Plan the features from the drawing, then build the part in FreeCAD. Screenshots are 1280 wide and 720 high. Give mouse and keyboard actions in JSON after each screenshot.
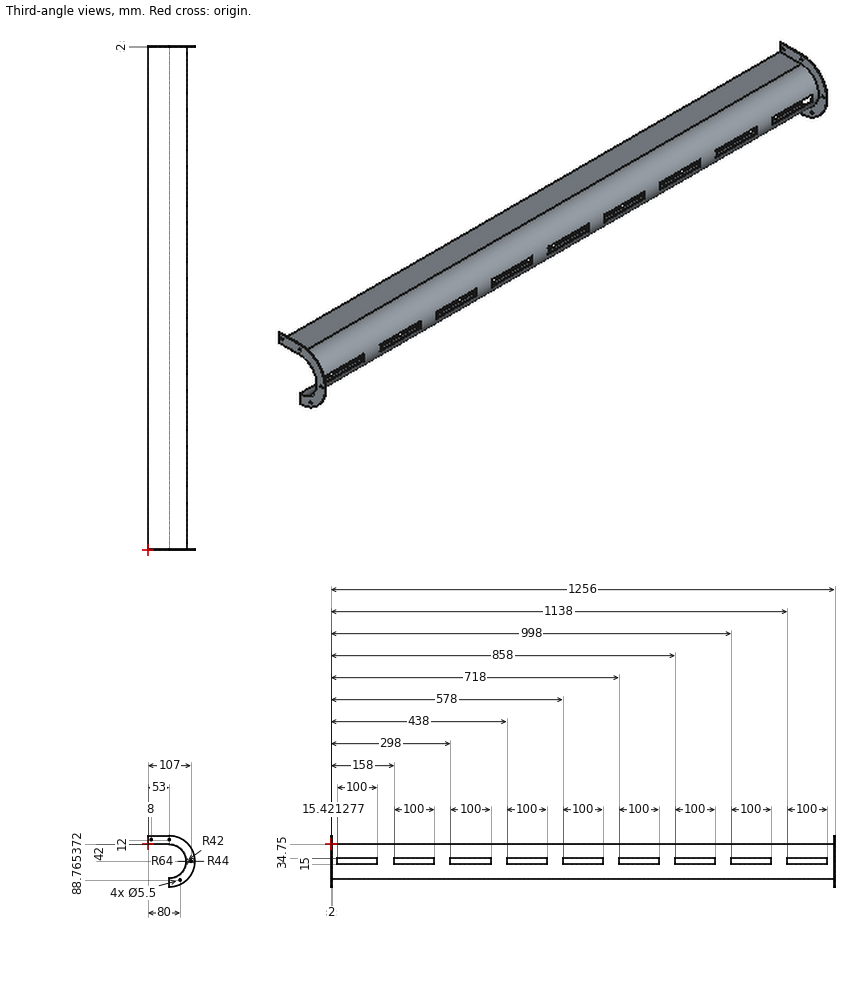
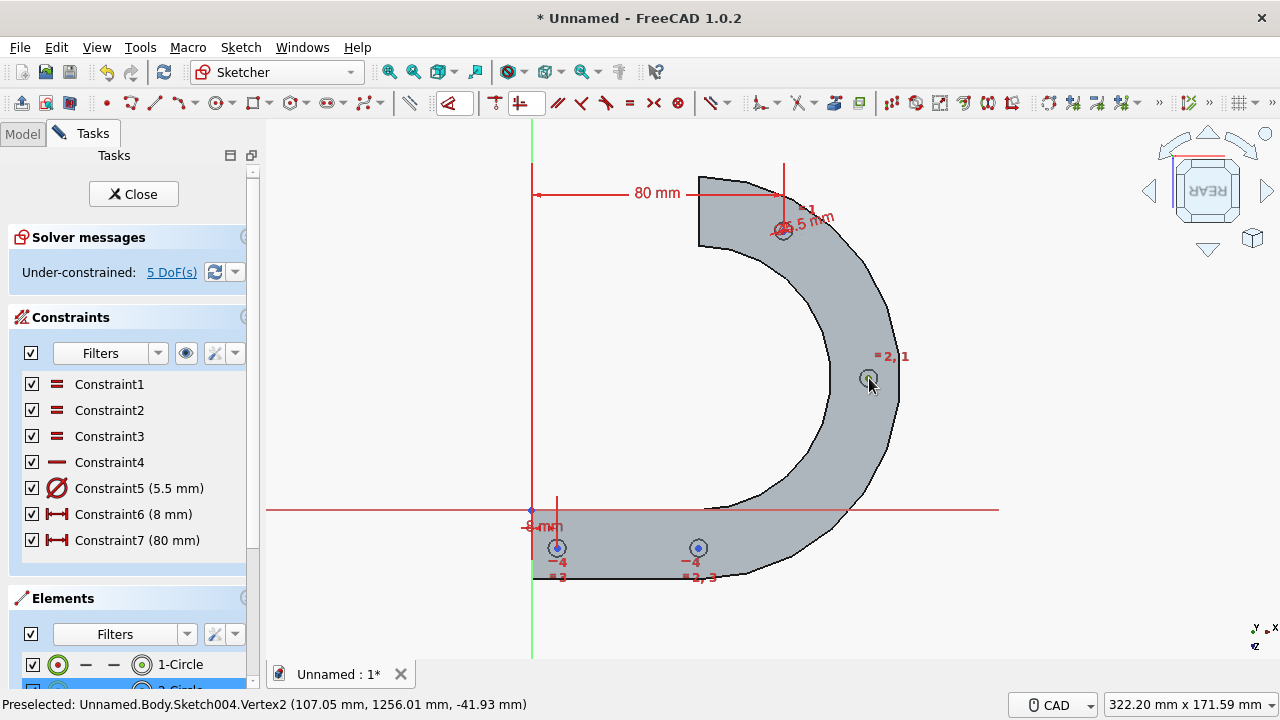
{"action": "key", "text": "i"}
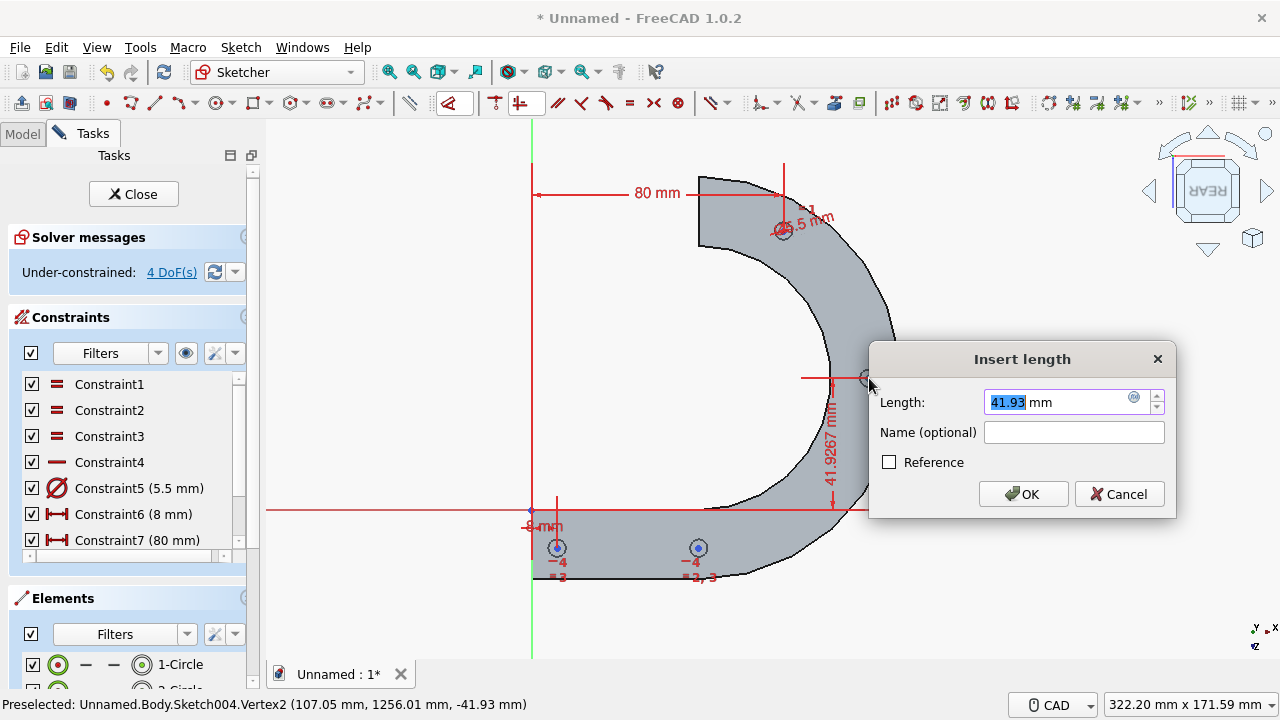
{"action": "type", "text": "42"}
{"action": "key", "text": "Return"}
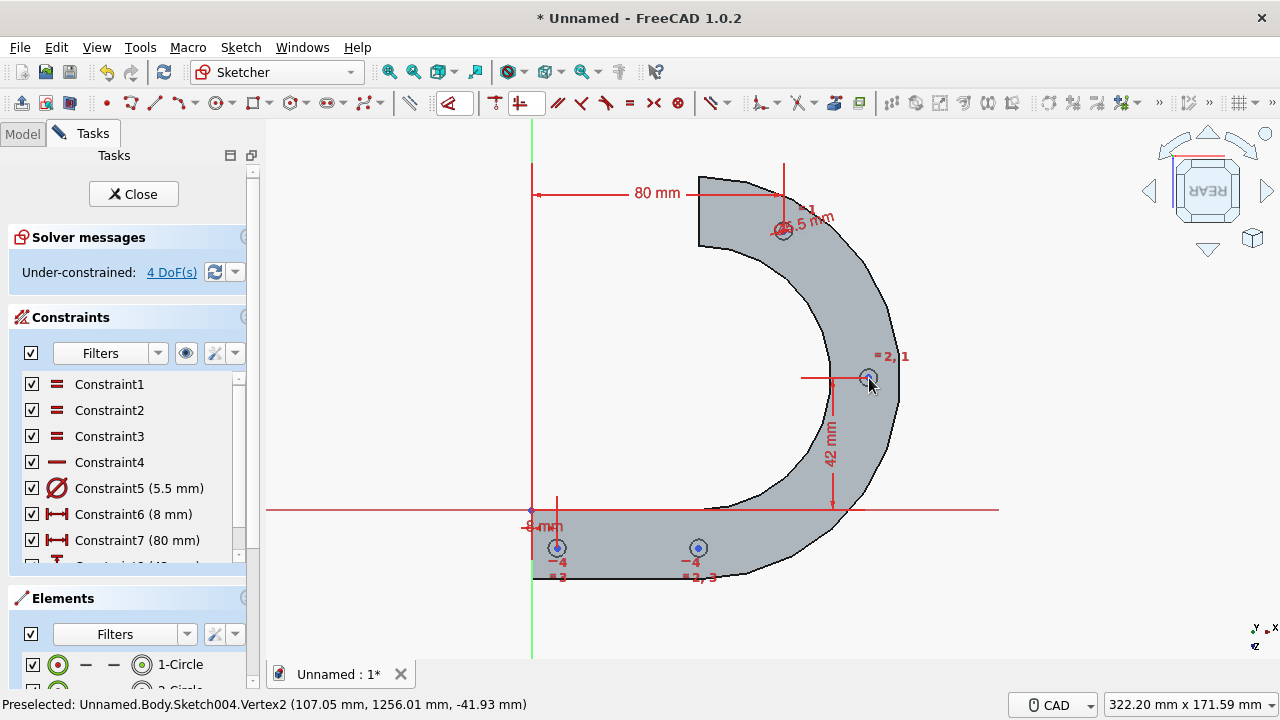
{"action": "left_click", "coordinate": [699, 548]}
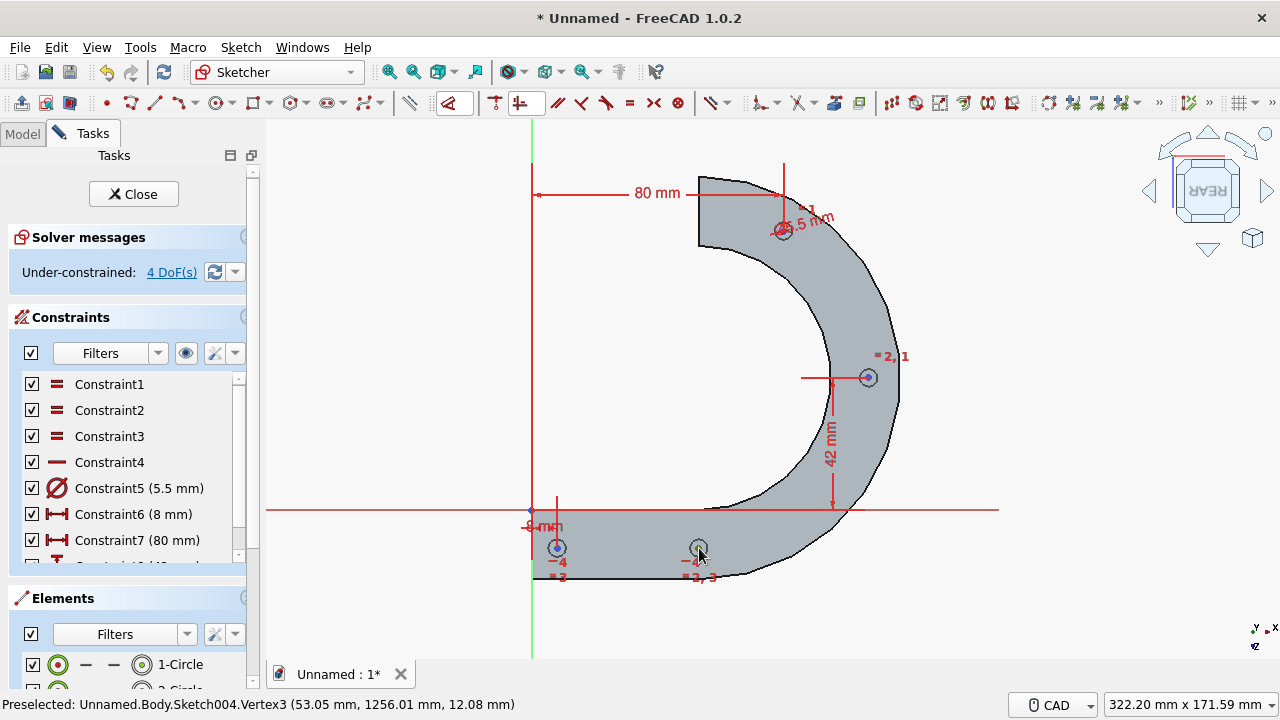
{"action": "left_click", "coordinate": [468, 104]}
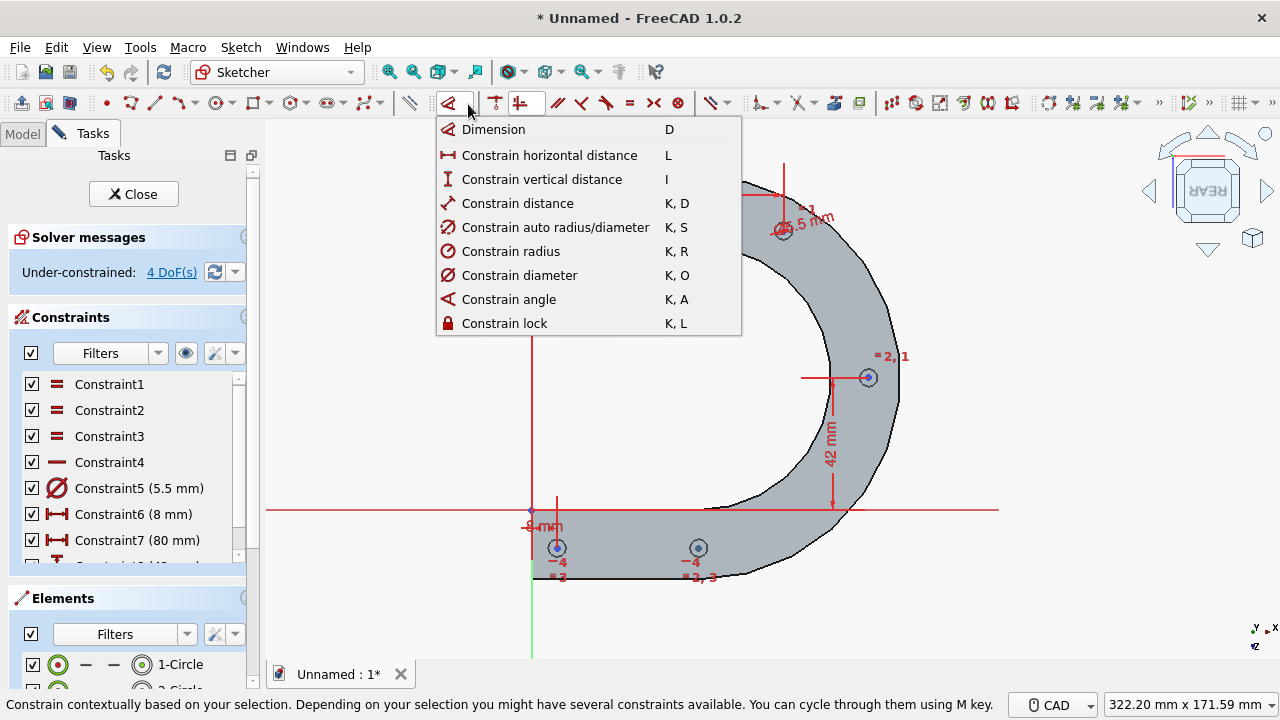
{"action": "left_click", "coordinate": [589, 155]}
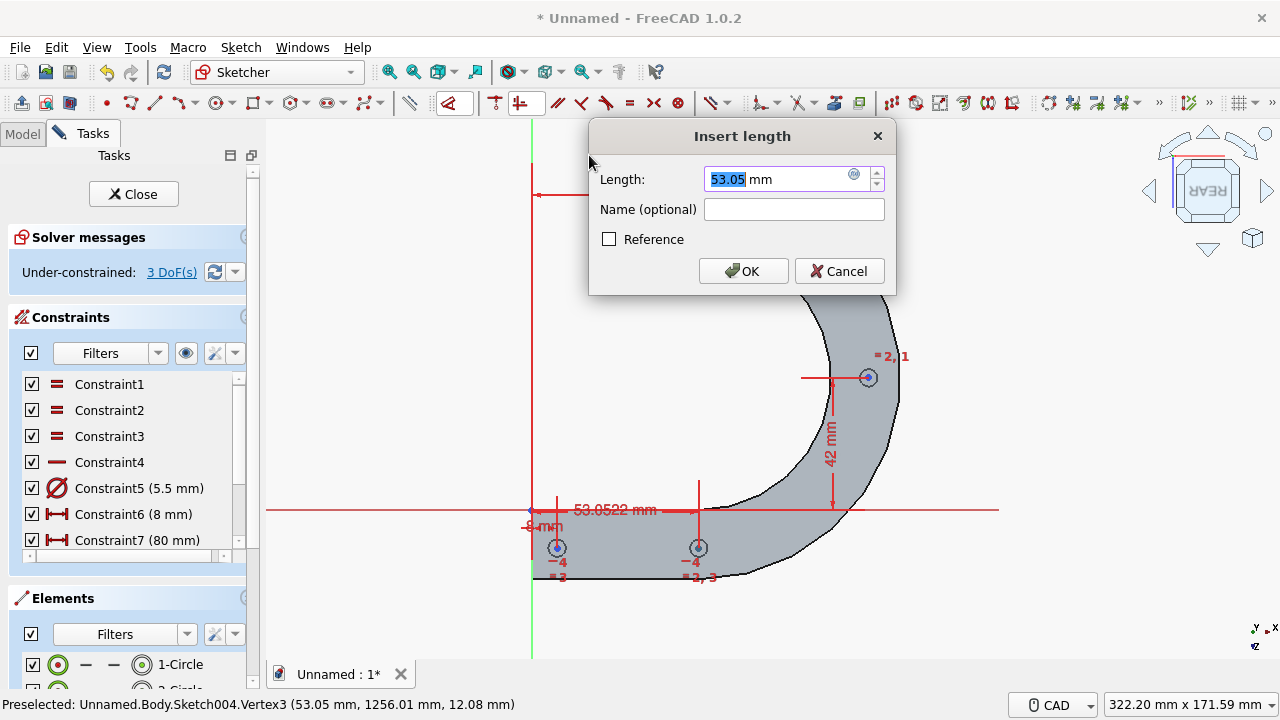
{"action": "type", "text": "53"}
{"action": "key", "text": "Return"}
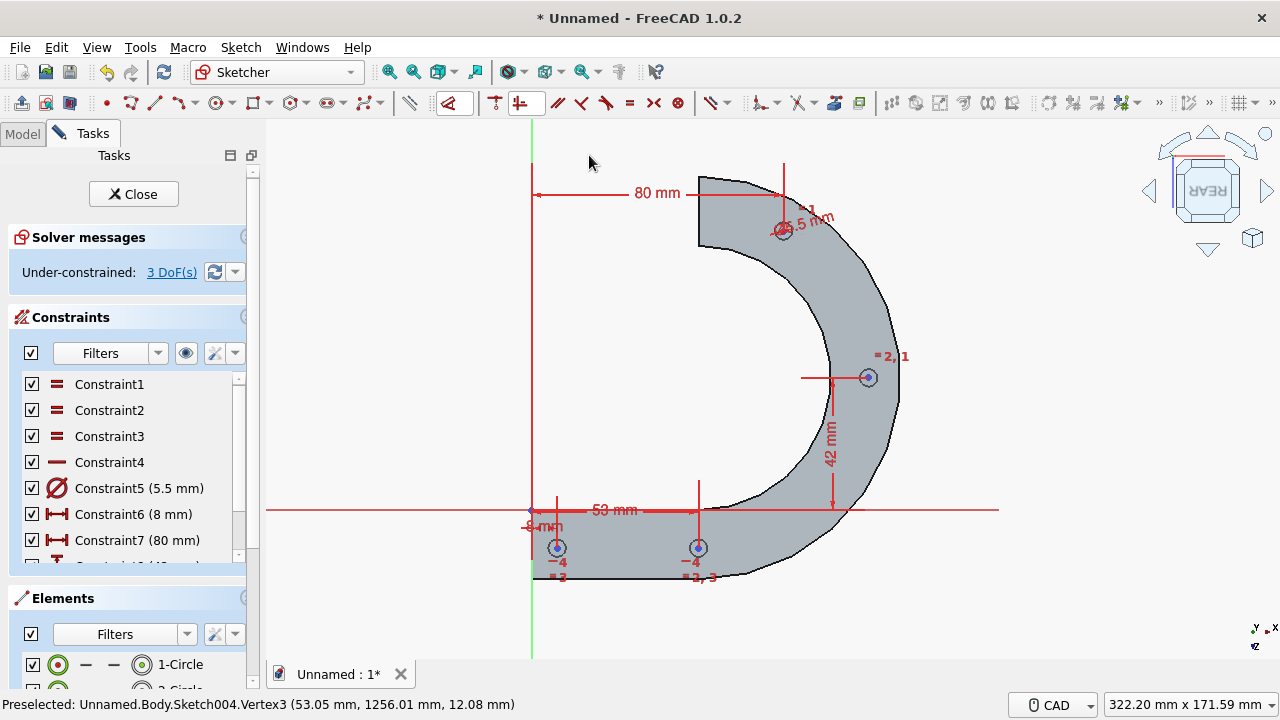
{"action": "left_click", "coordinate": [699, 548]}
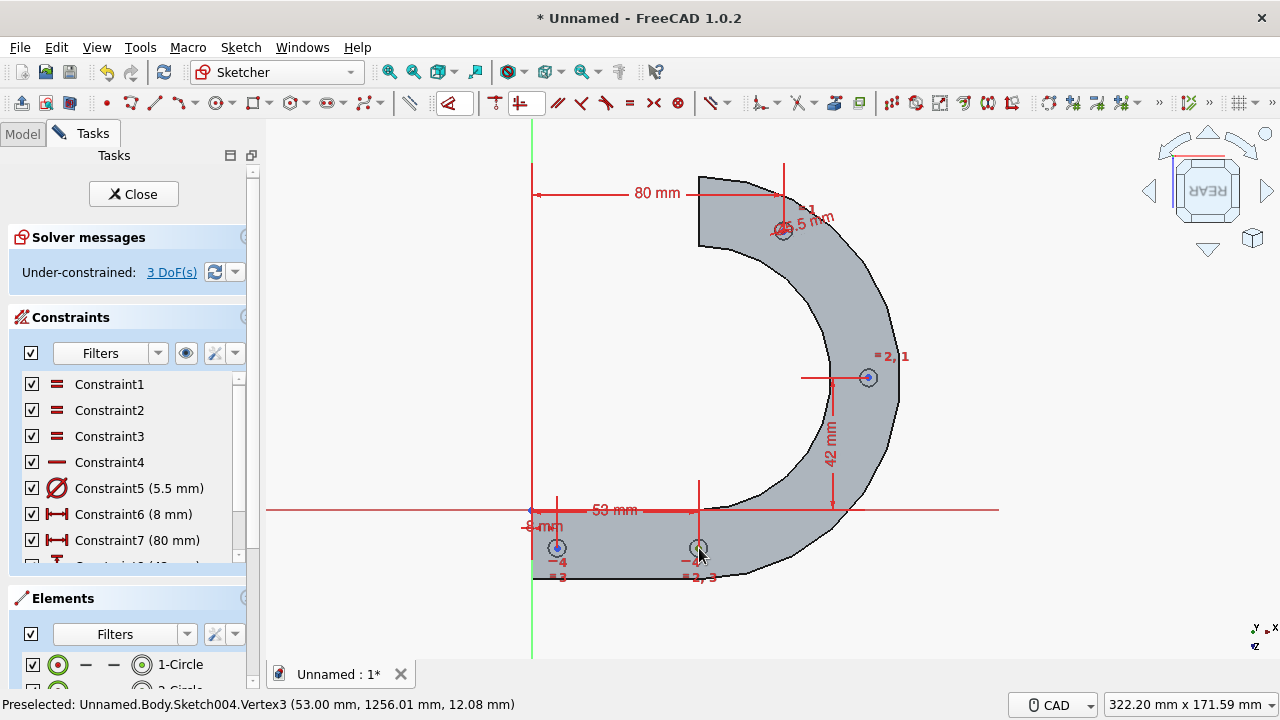
{"action": "key", "text": "i"}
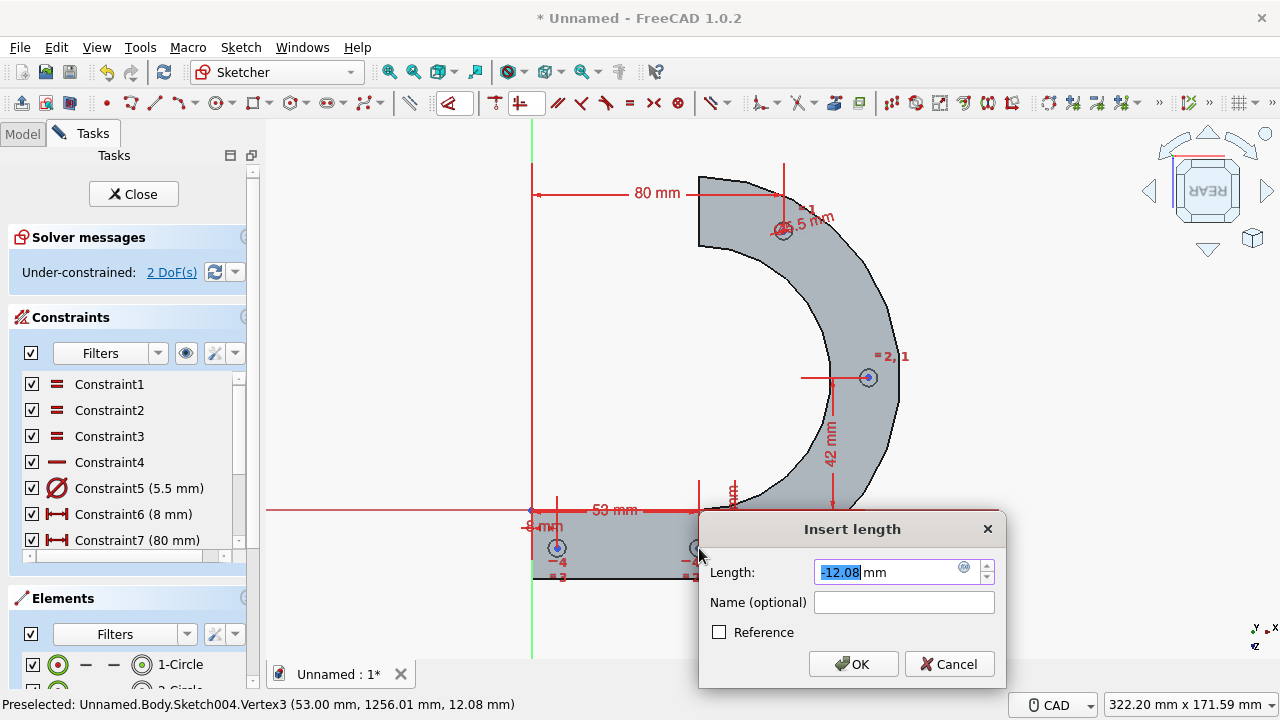
{"action": "type", "text": "-12"}
{"action": "key", "text": "Return"}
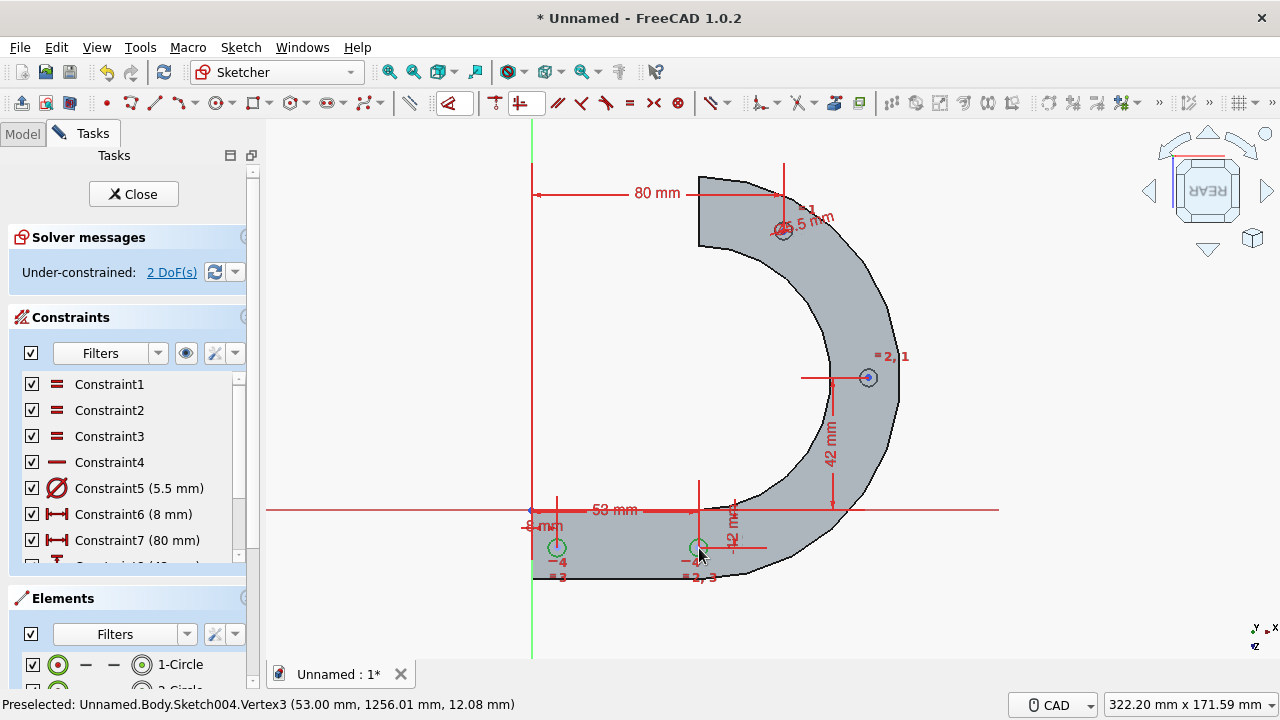
{"action": "left_click", "coordinate": [869, 378]}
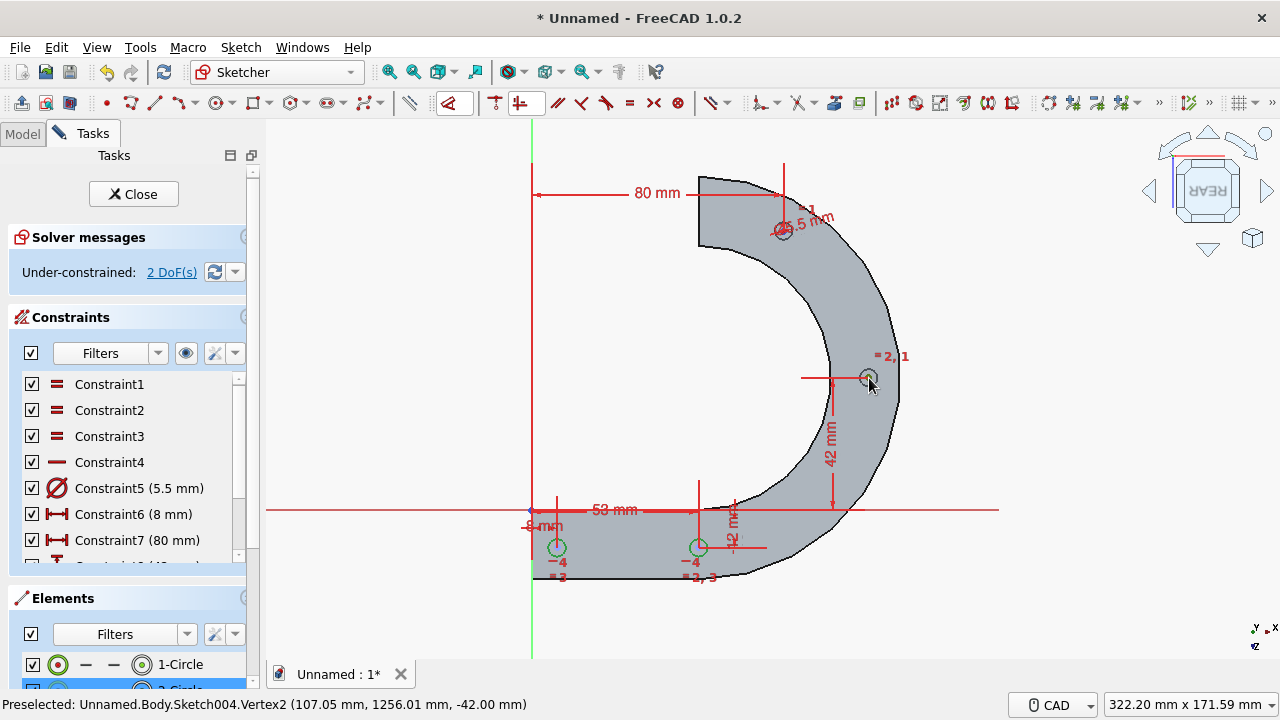
{"action": "left_click", "coordinate": [468, 104]}